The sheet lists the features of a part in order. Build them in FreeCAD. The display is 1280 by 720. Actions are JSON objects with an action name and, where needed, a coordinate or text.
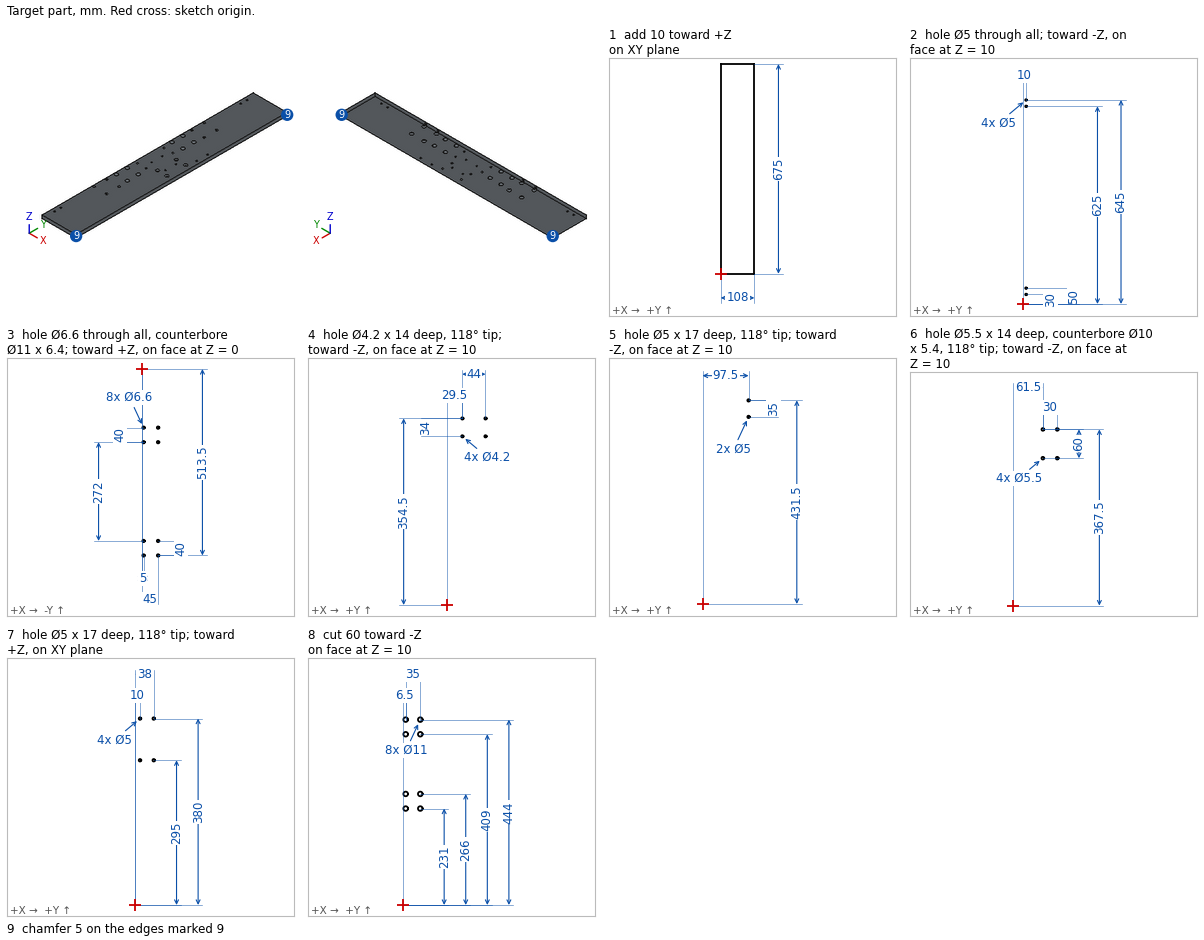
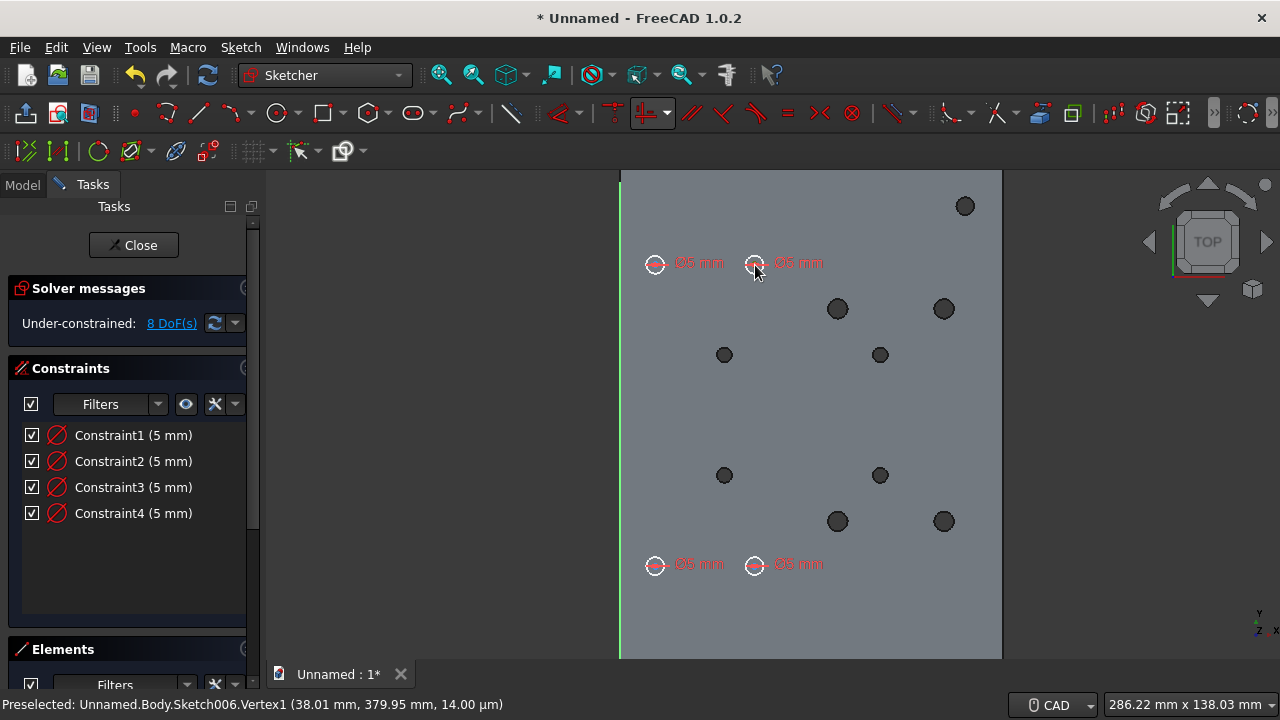
{"action": "left_click", "coordinate": [655, 265]}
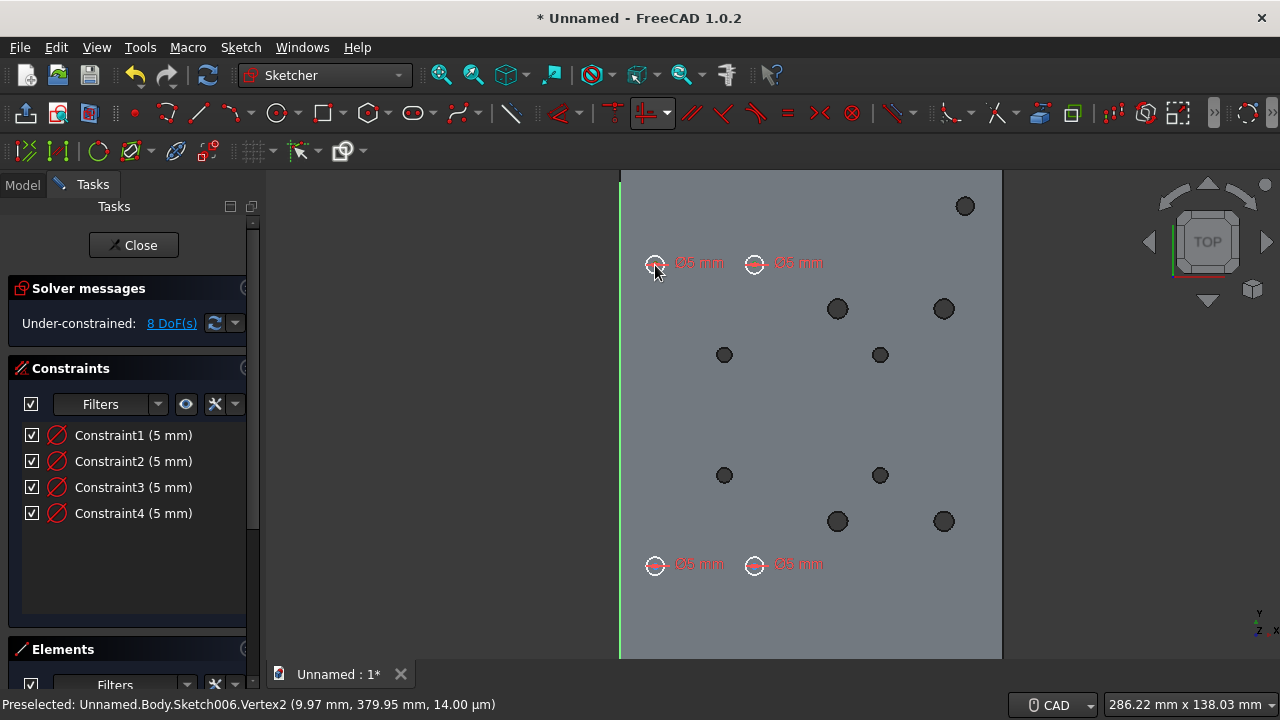
{"action": "left_click", "coordinate": [670, 114]}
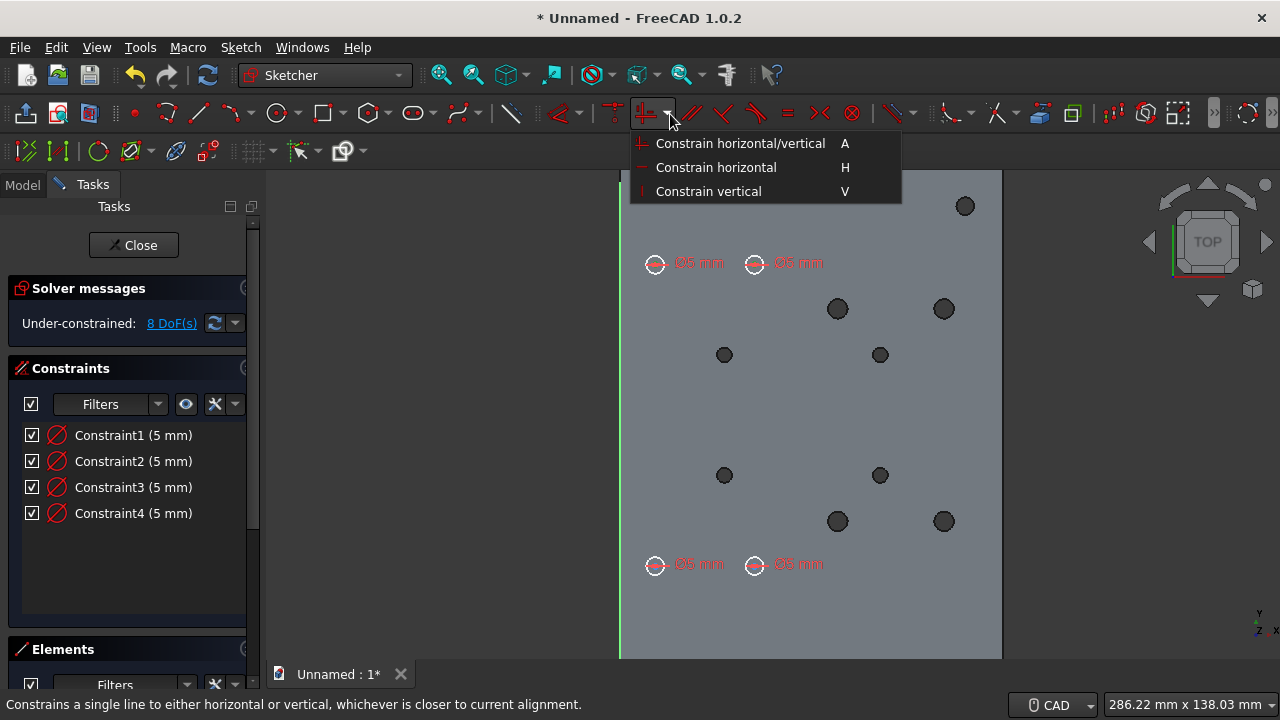
{"action": "left_click", "coordinate": [766, 167]}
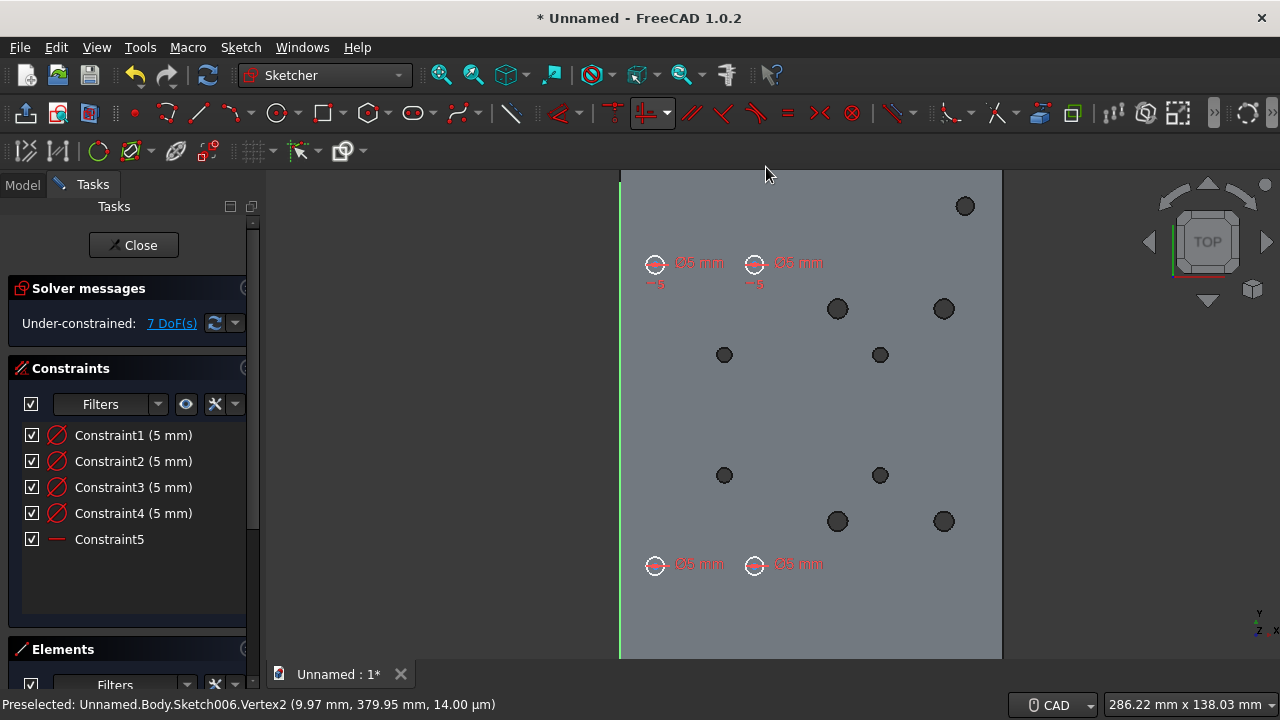
{"action": "left_click", "coordinate": [755, 265]}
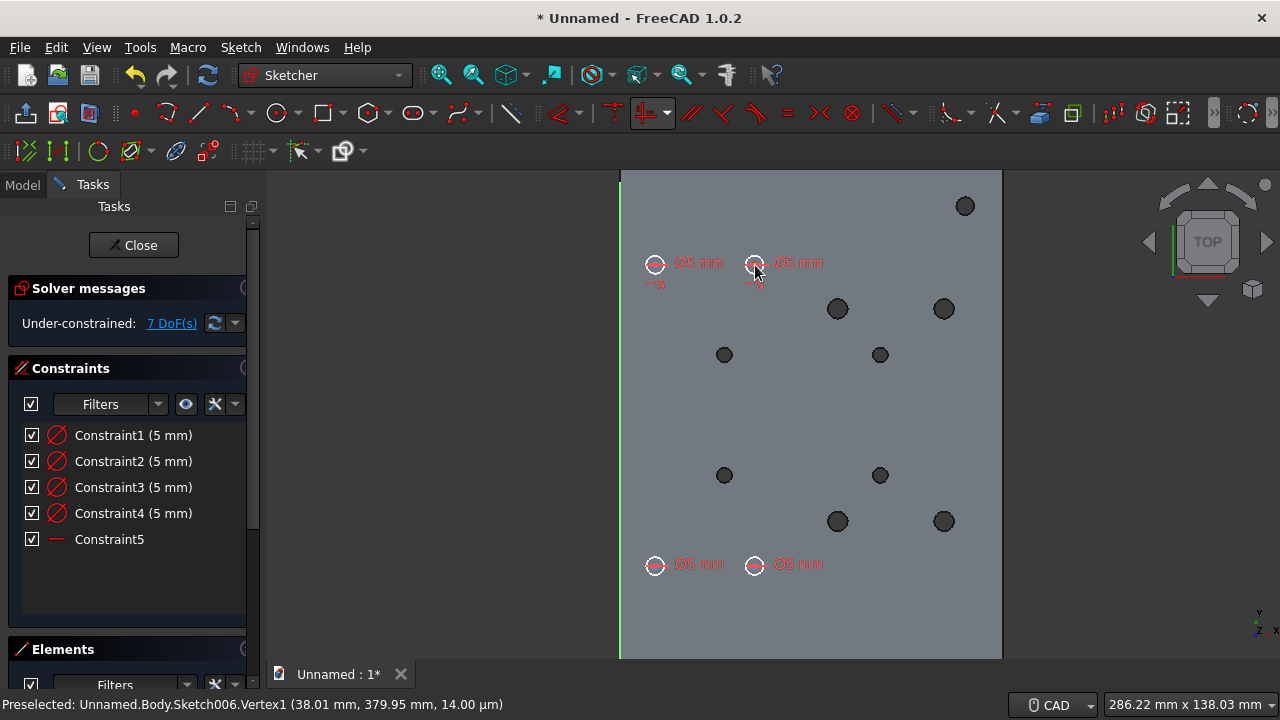
{"action": "left_click", "coordinate": [755, 566]}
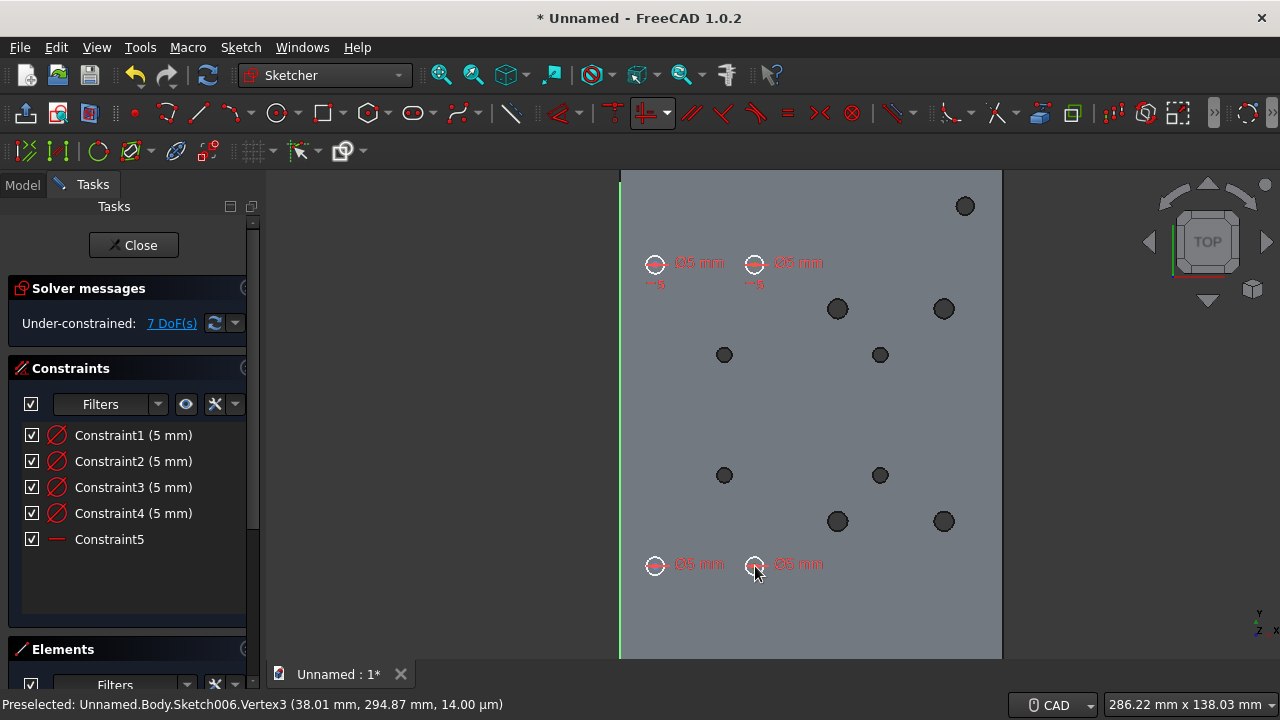
{"action": "key", "text": "v"}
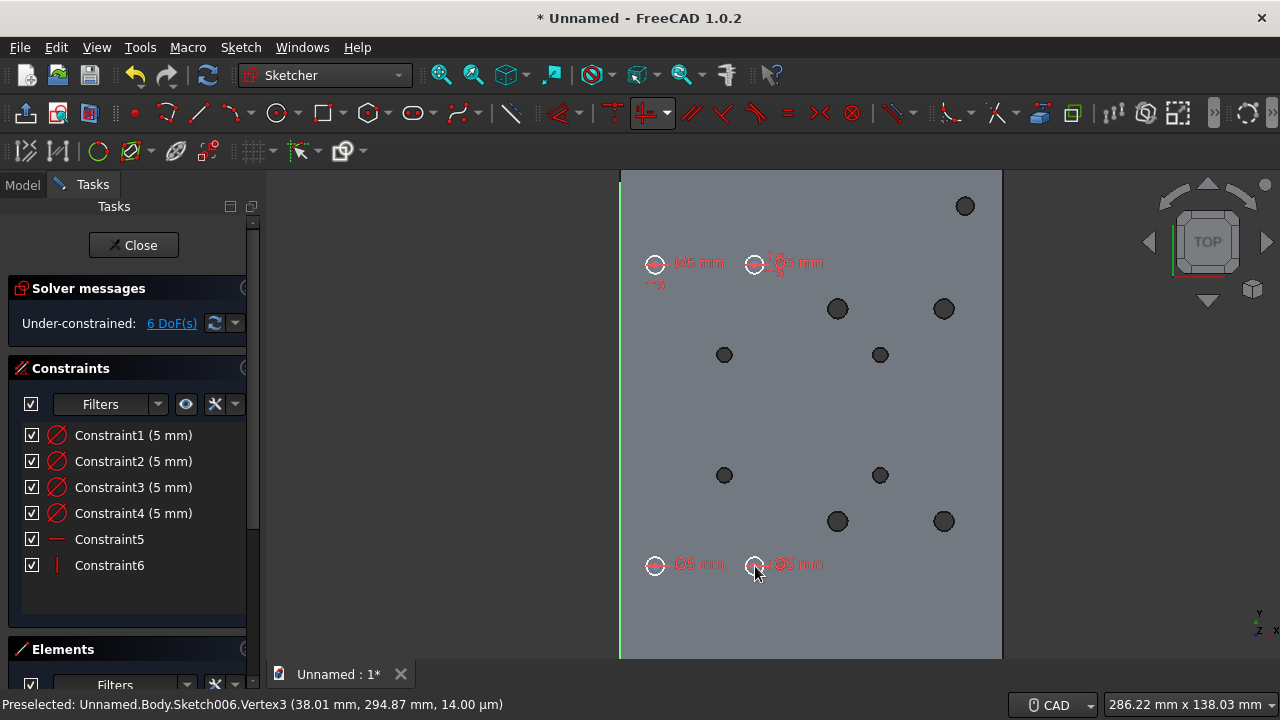
{"action": "left_click", "coordinate": [655, 265]}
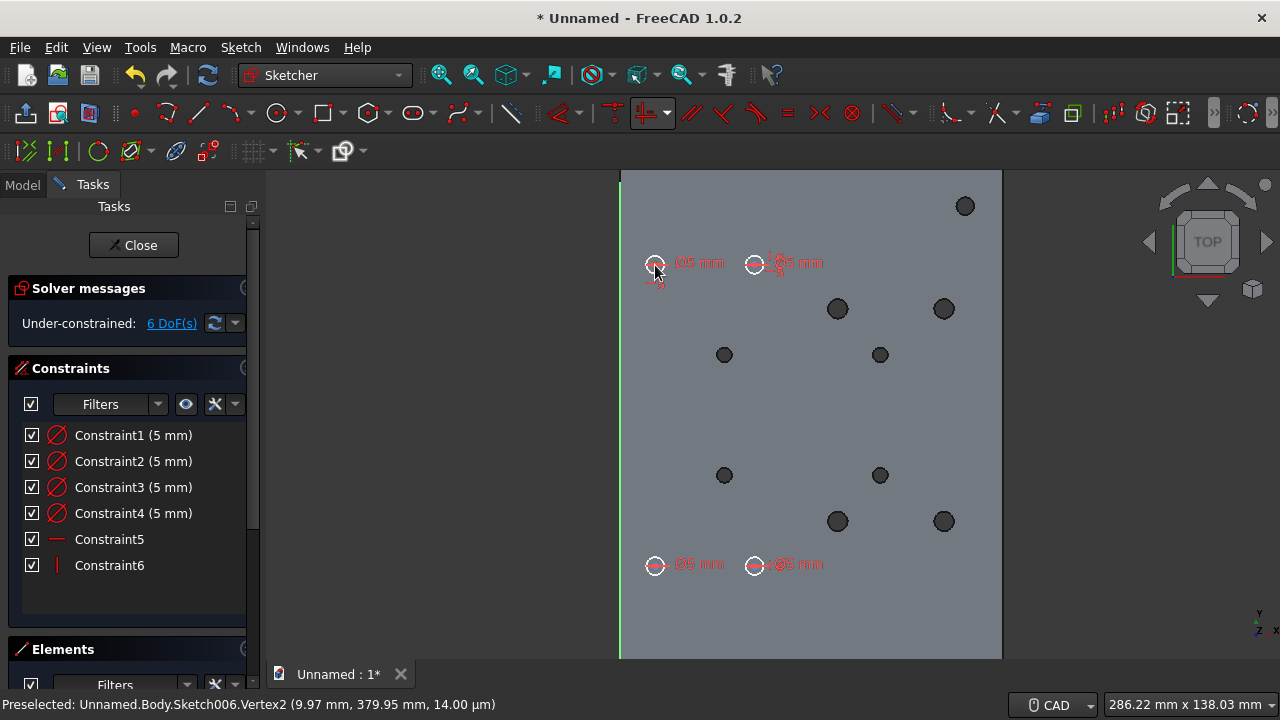
{"action": "left_click", "coordinate": [655, 566]}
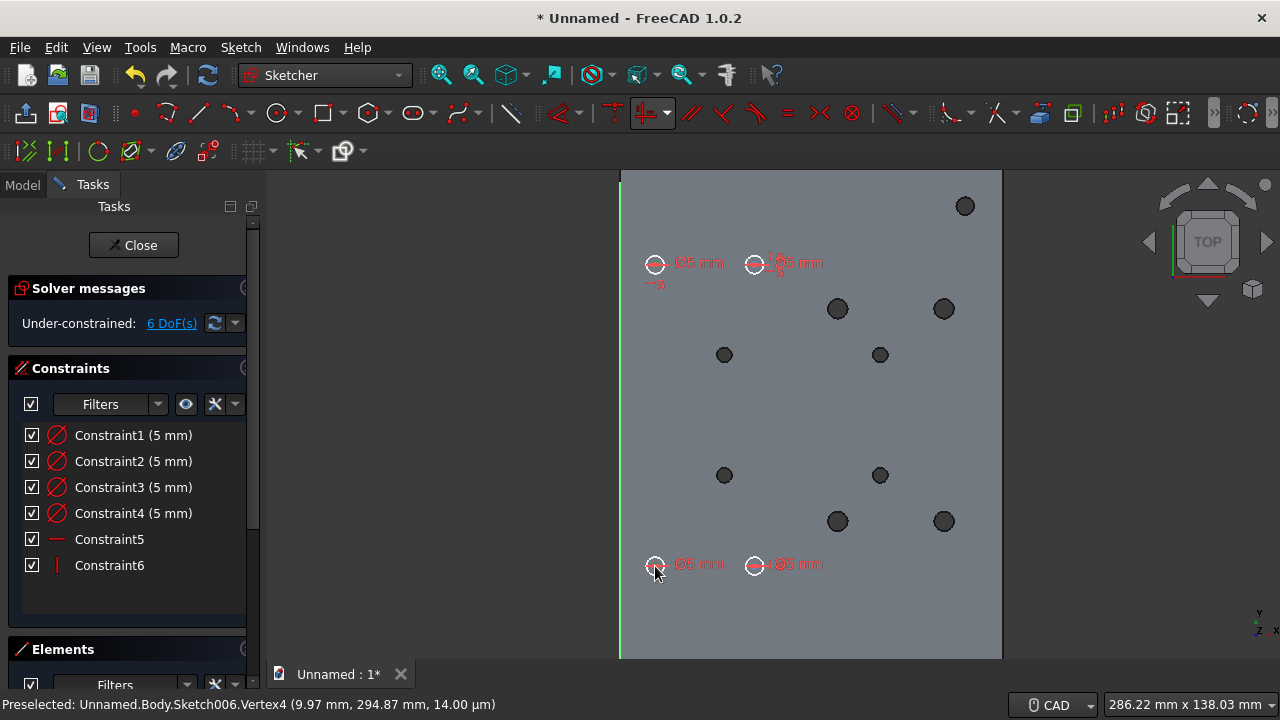
{"action": "key", "text": "v"}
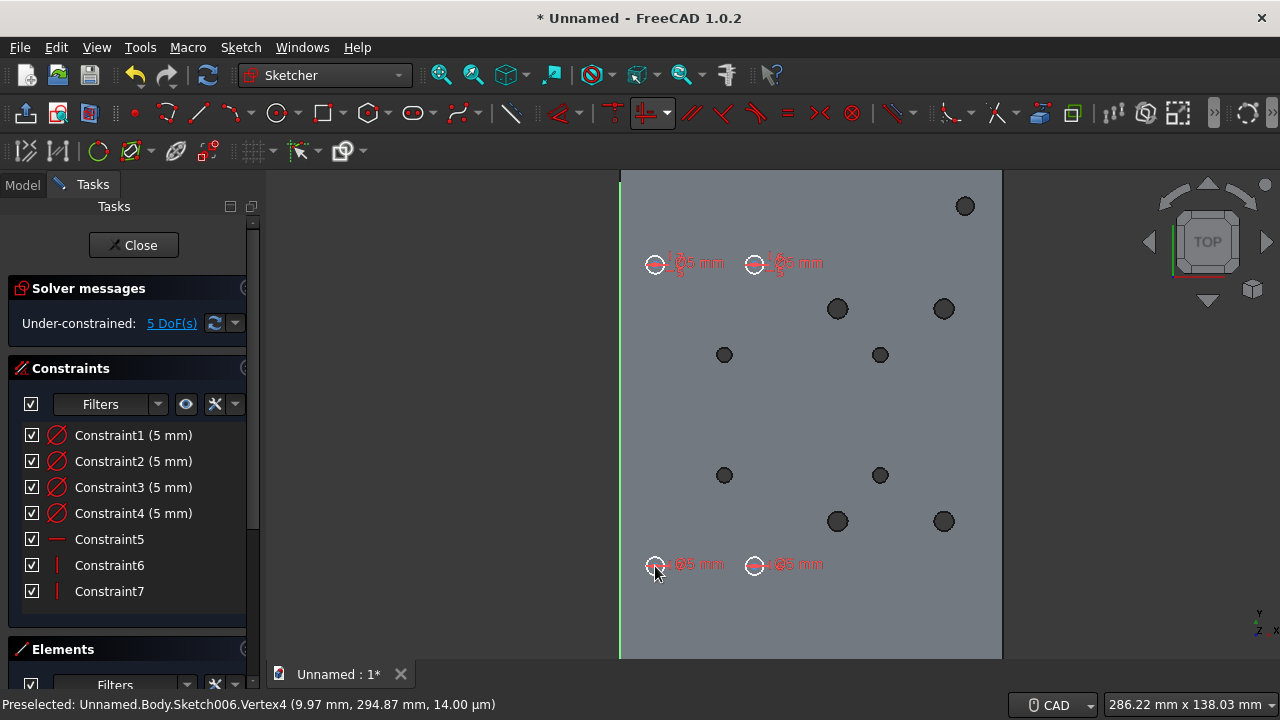
{"action": "left_click", "coordinate": [755, 566]}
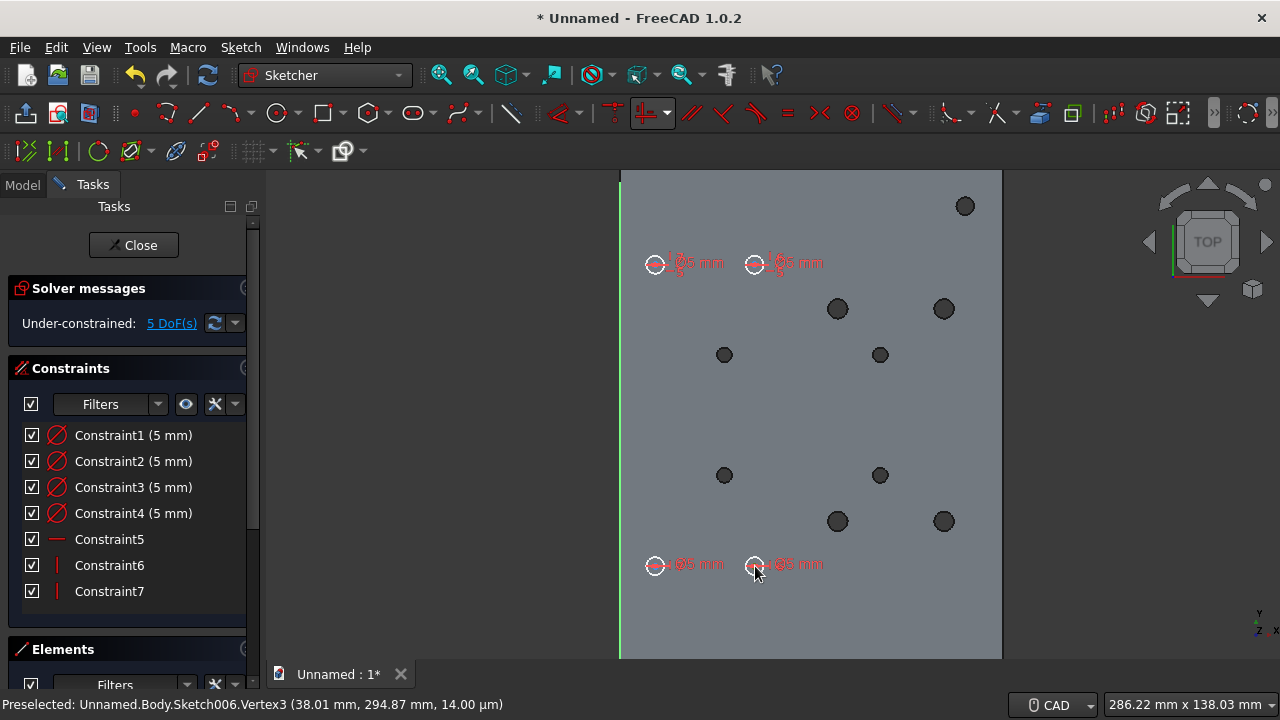
{"action": "left_click", "coordinate": [655, 566]}